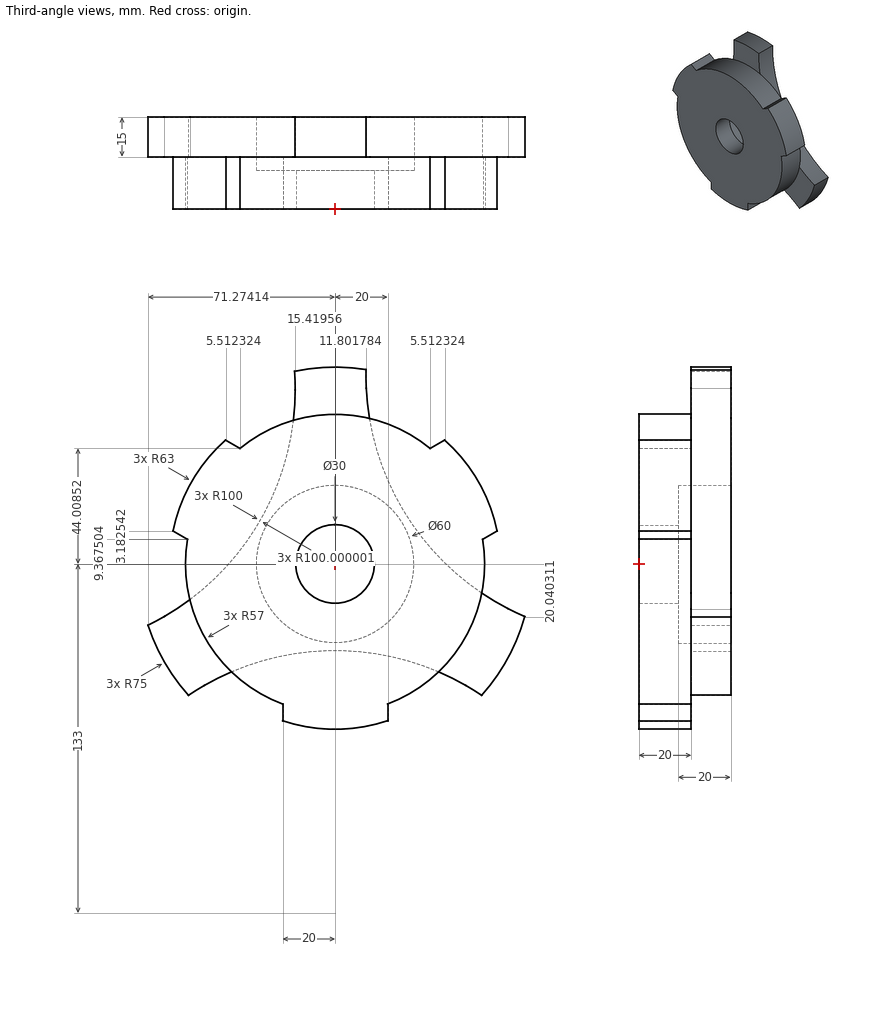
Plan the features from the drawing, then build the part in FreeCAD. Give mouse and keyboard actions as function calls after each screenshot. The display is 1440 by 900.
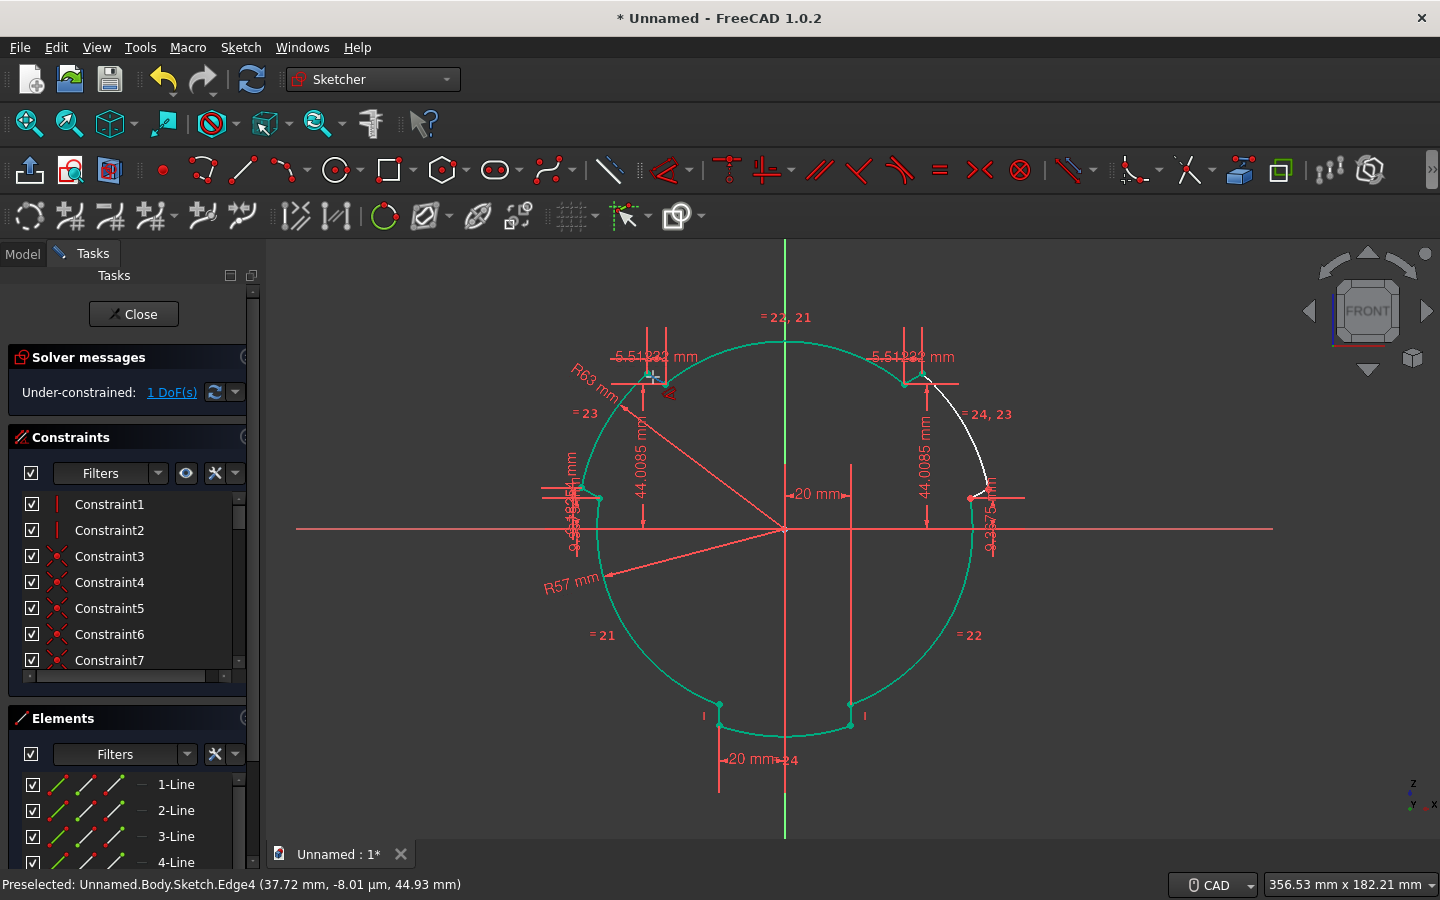
scroll(983, 492, up, 7)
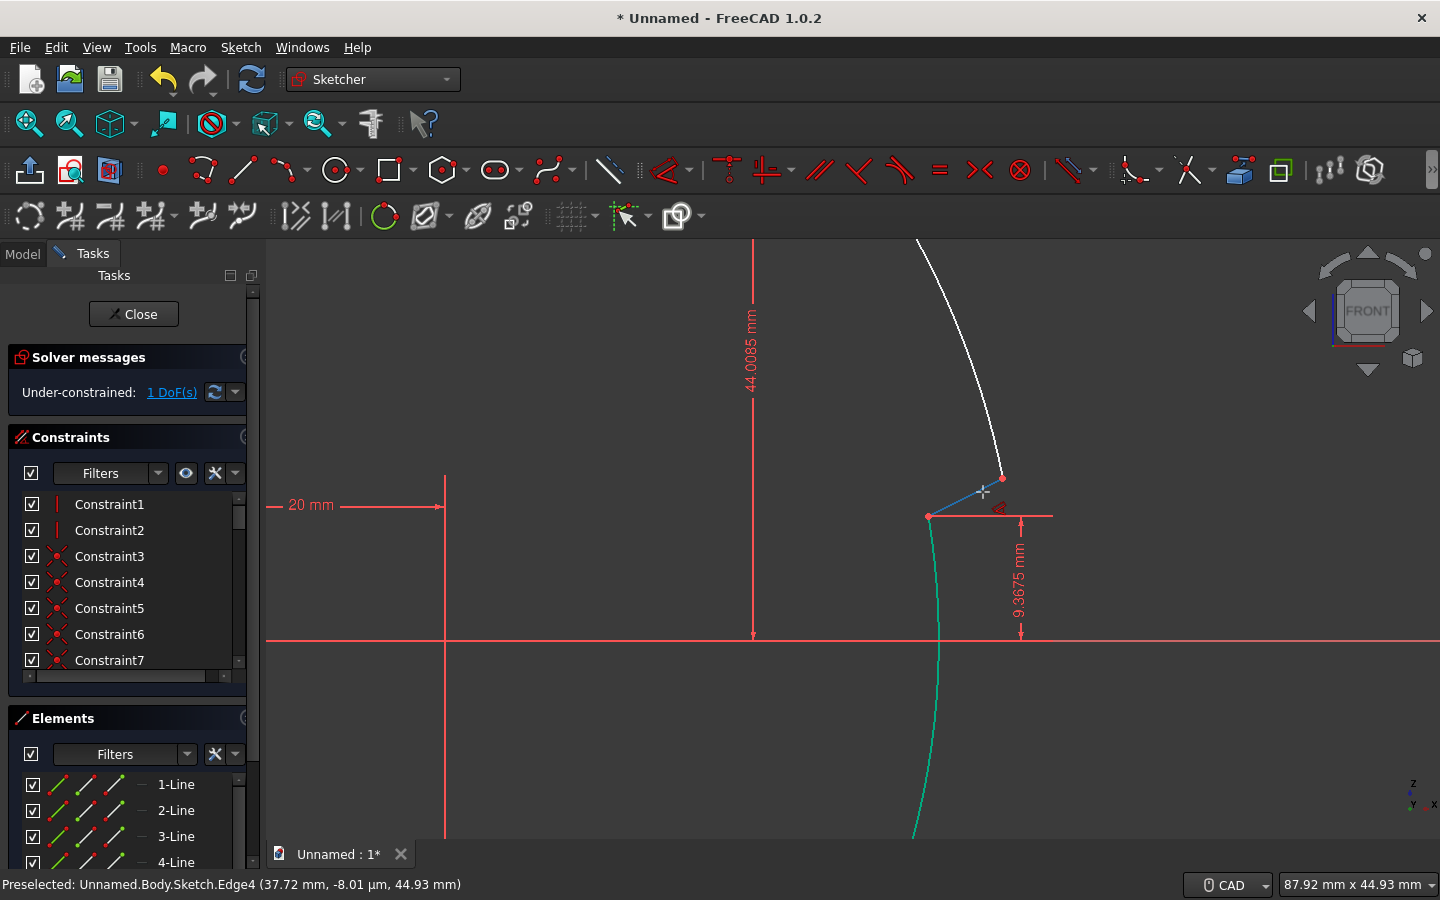
click(981, 490)
click(1037, 497)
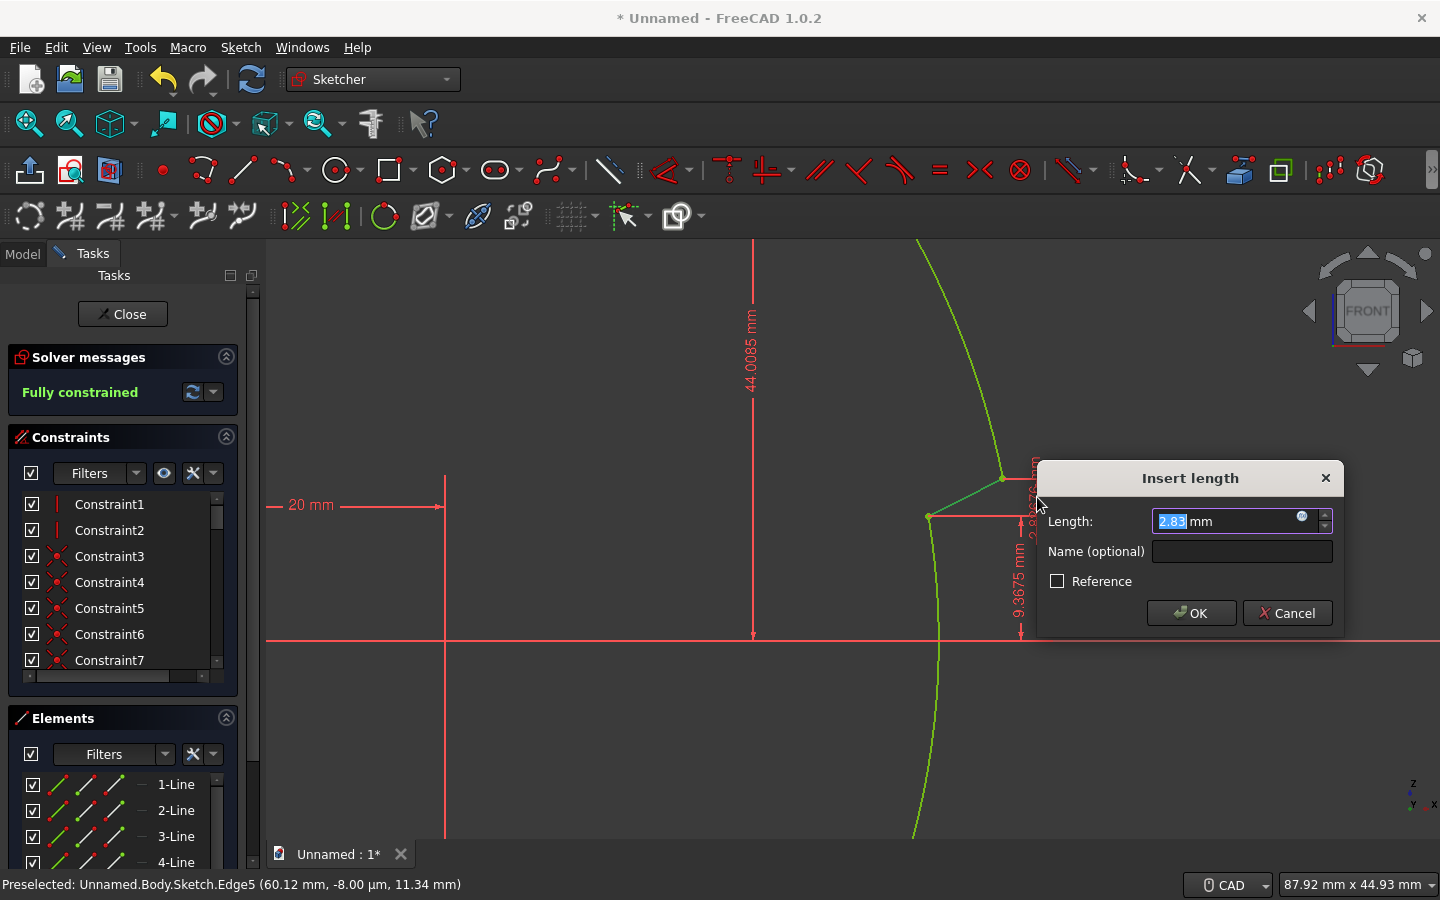
text(3.182542)
key(Return)
key(Escape)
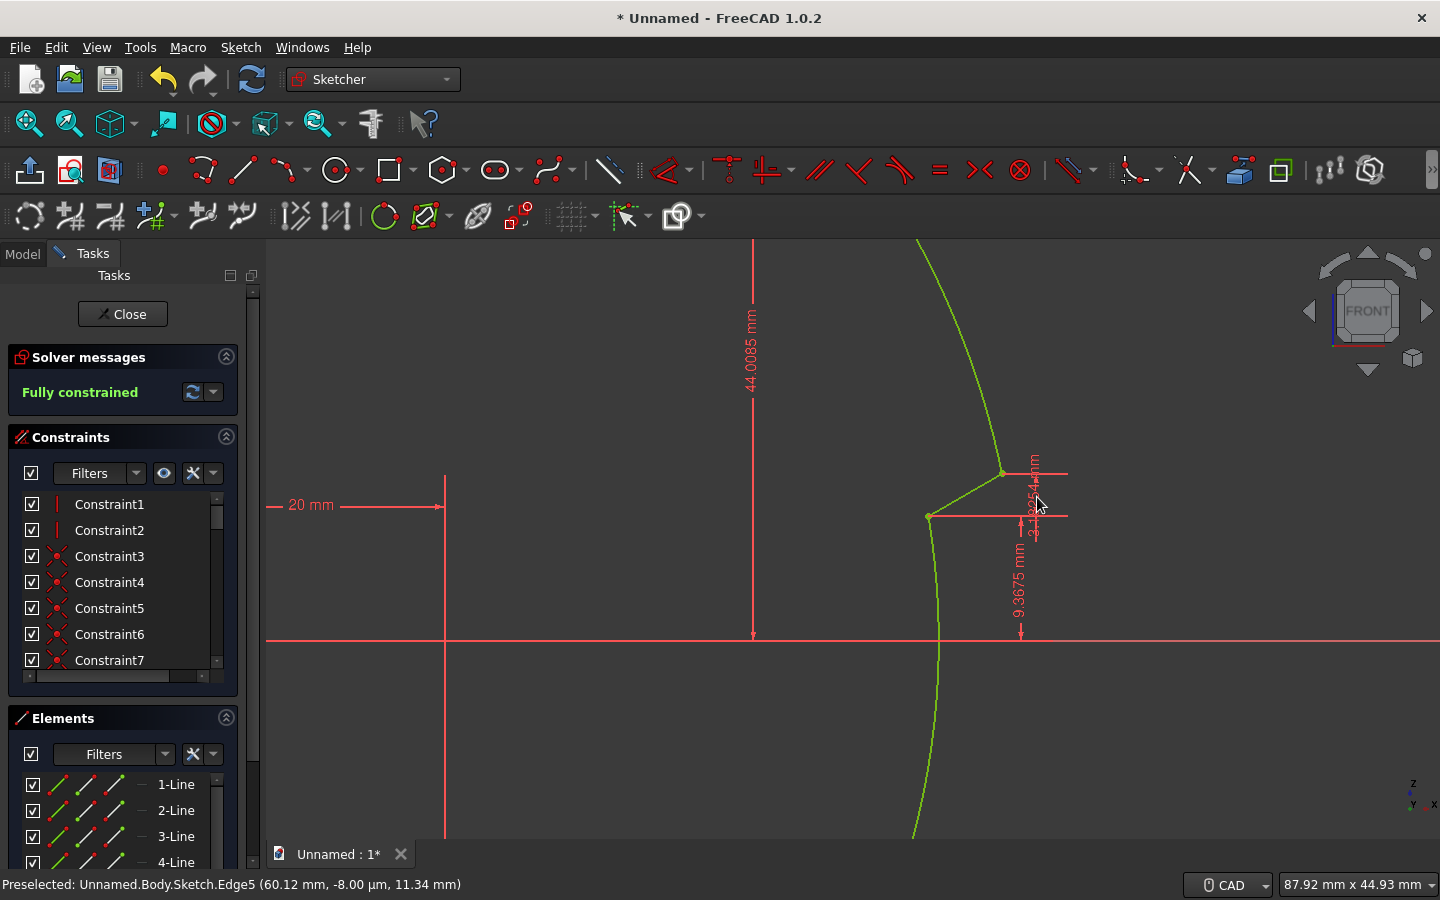
click(123, 314)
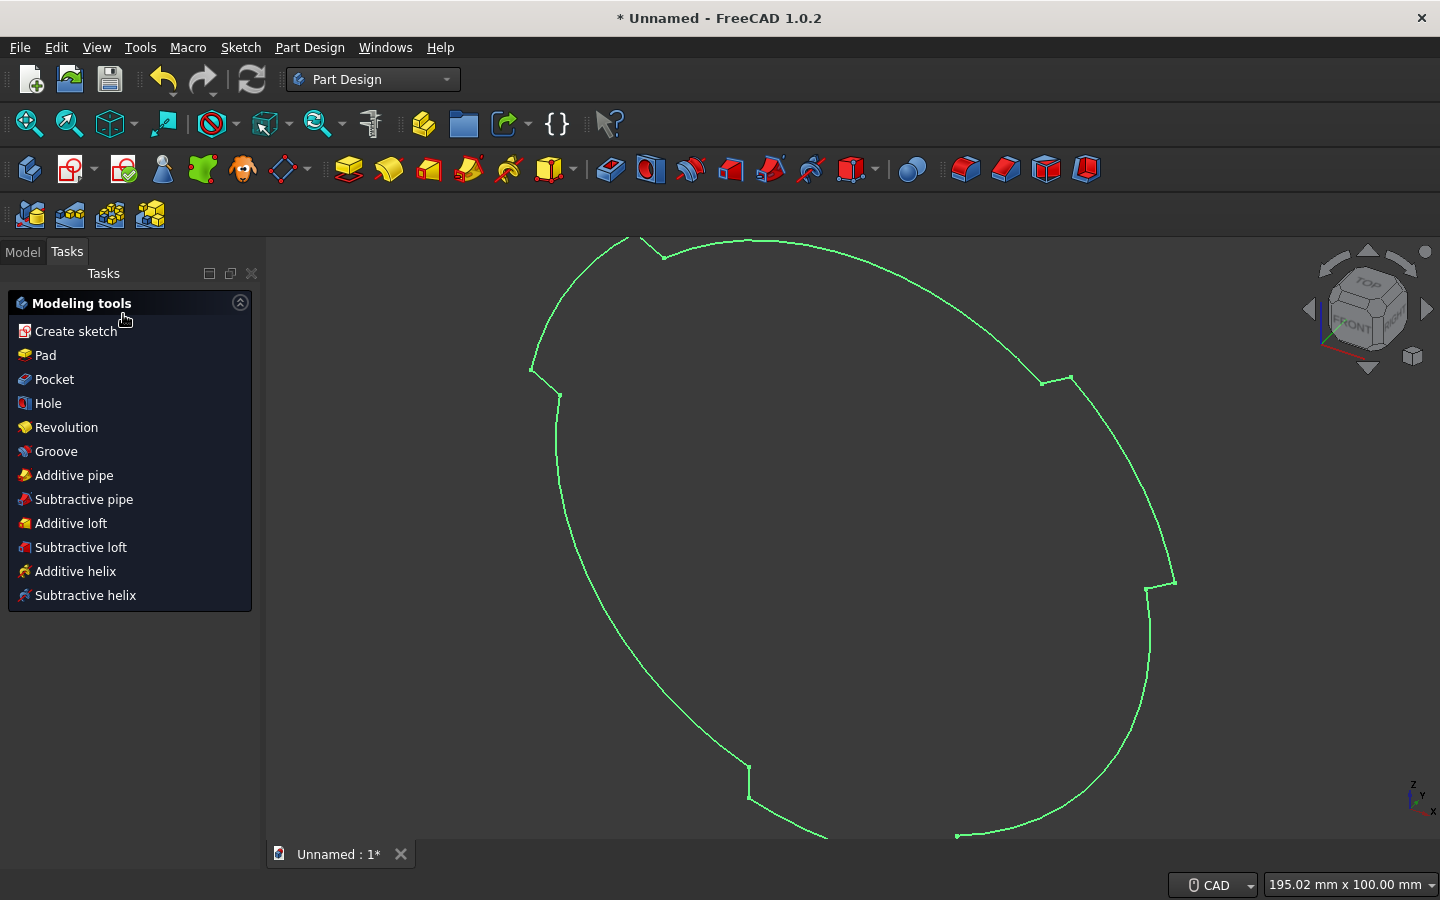
click(350, 170)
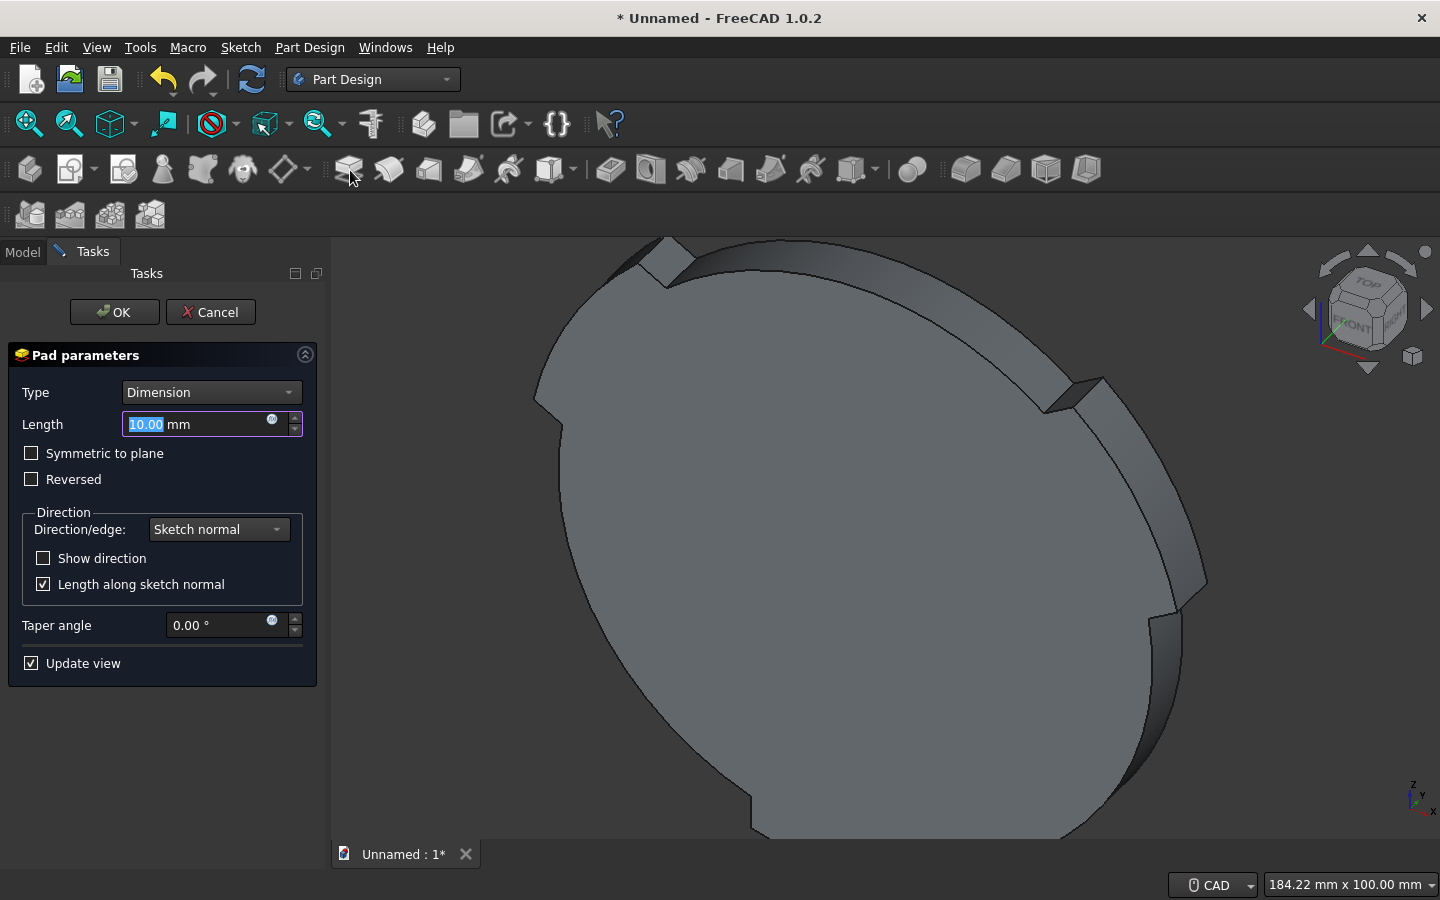
text(20)
key(Tab)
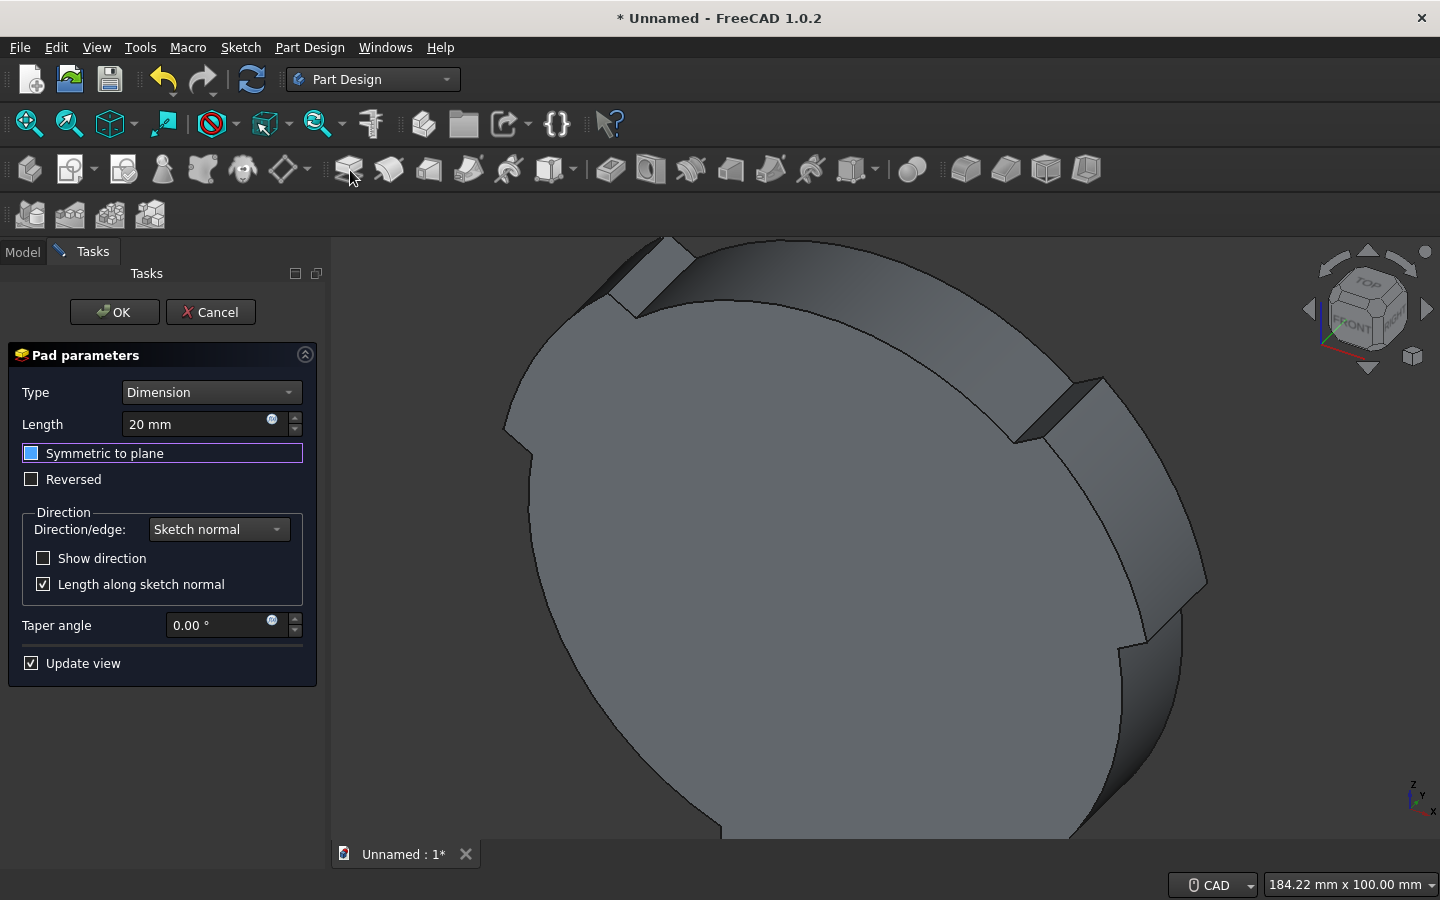
click(30, 479)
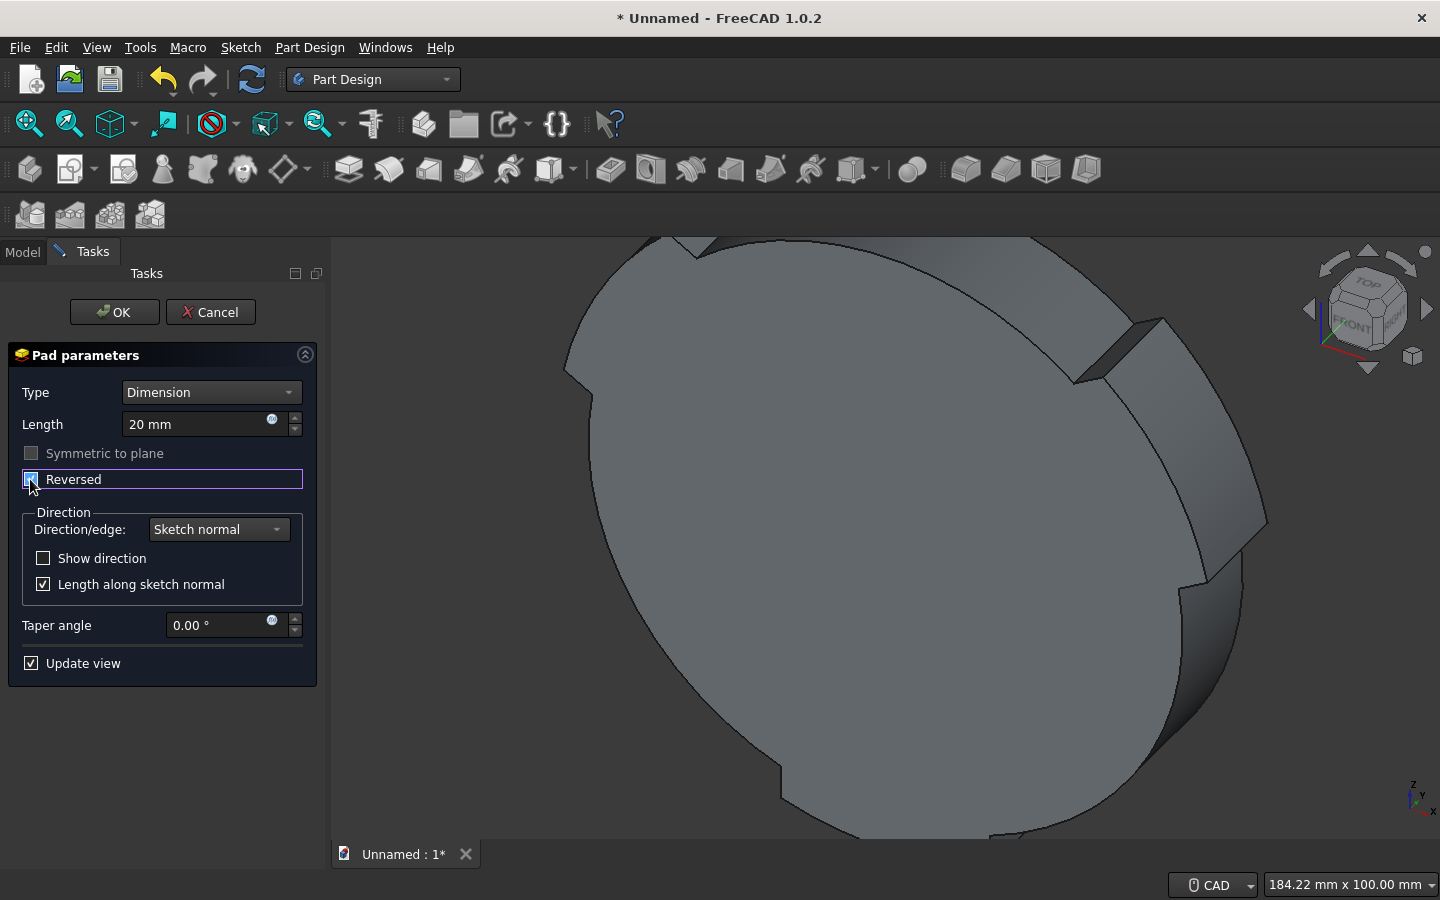
click(115, 312)